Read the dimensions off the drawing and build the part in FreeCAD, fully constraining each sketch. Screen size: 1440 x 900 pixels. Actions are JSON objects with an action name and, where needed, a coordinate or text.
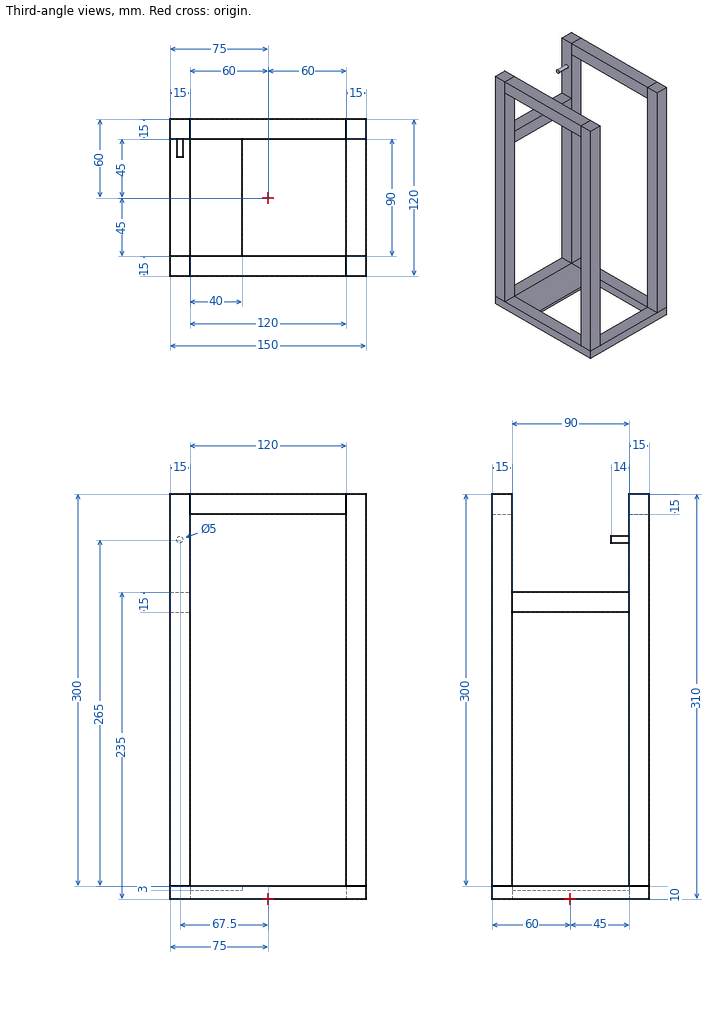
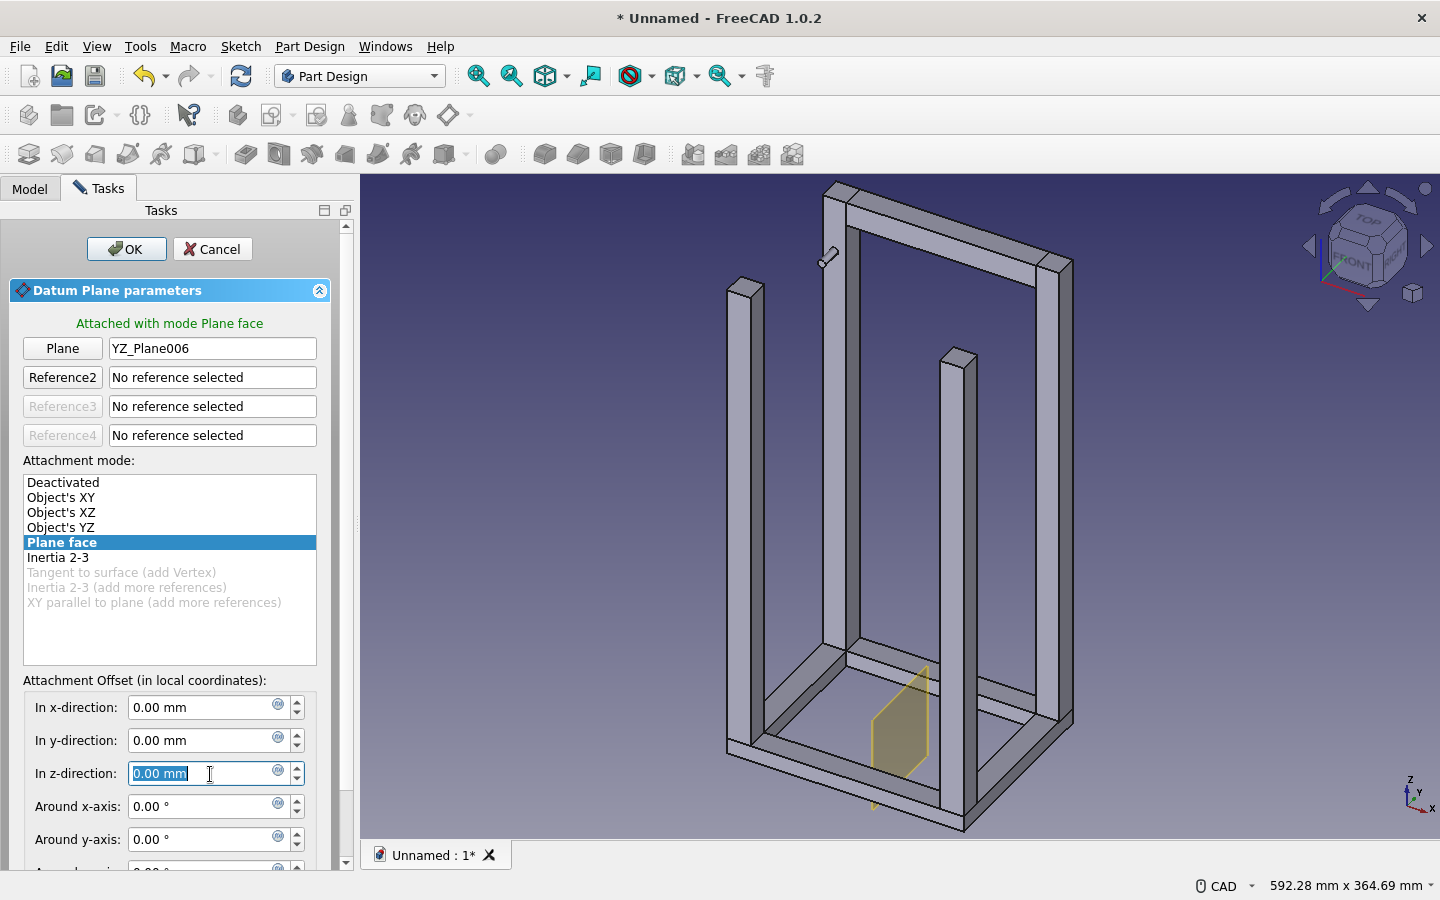
{"action": "type", "text": "-60"}
{"action": "key", "text": "Tab"}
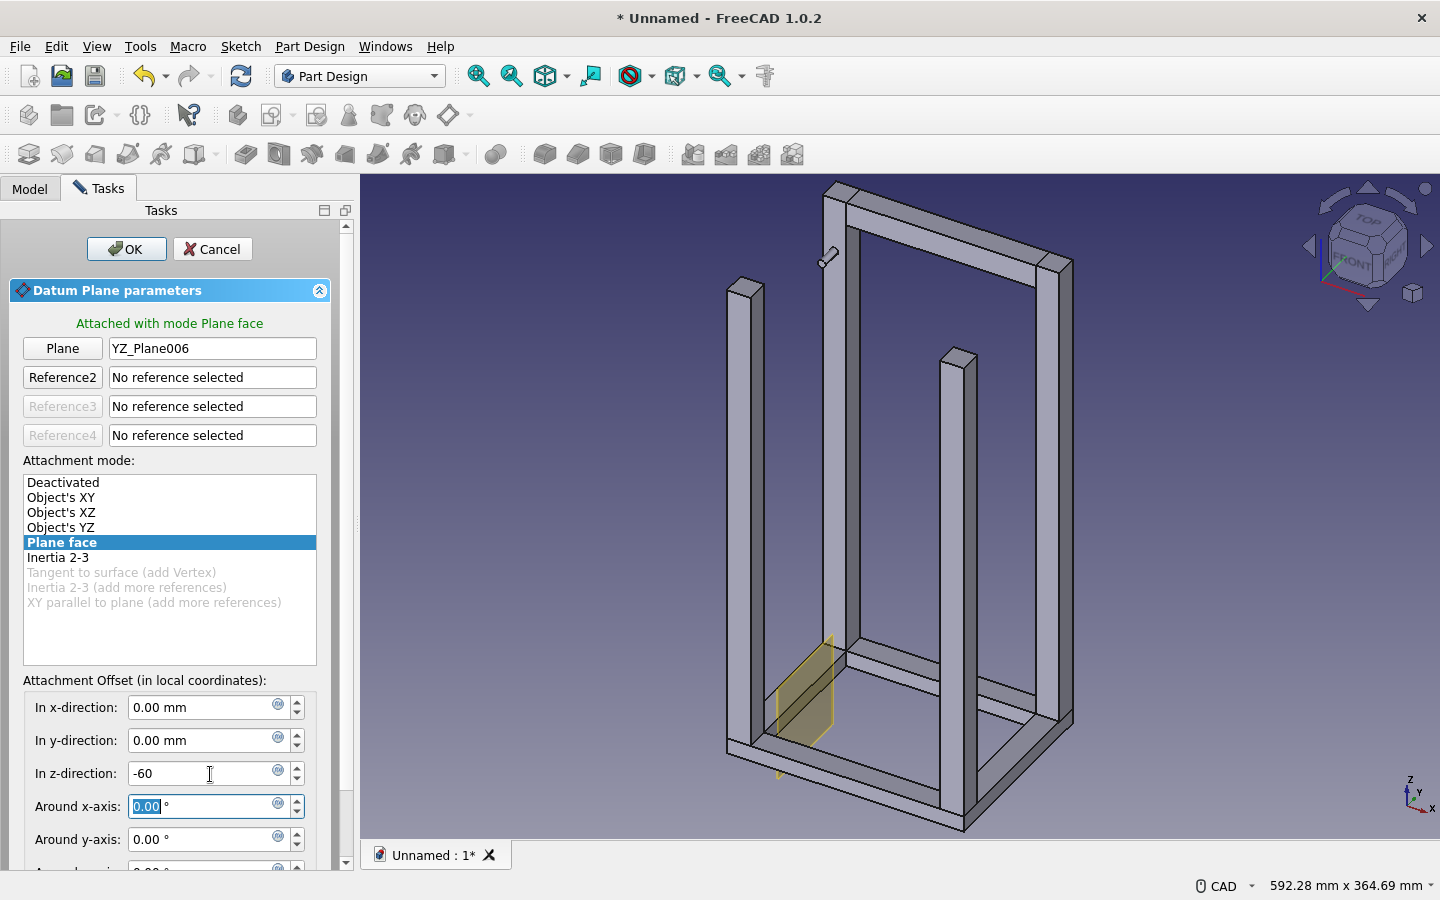
{"action": "left_click", "coordinate": [127, 249]}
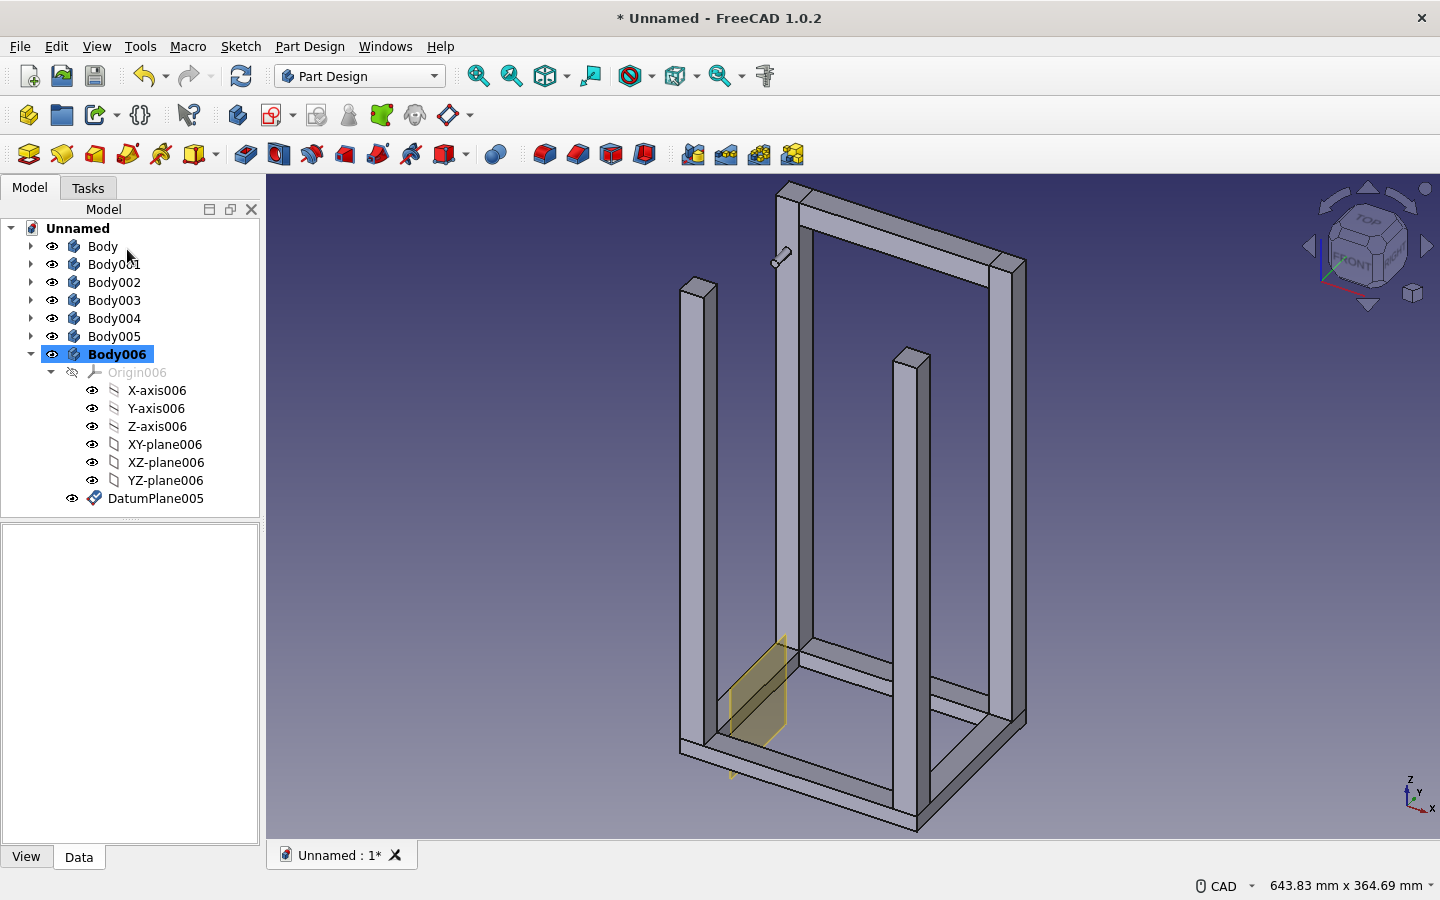
{"action": "left_click", "coordinate": [117, 498]}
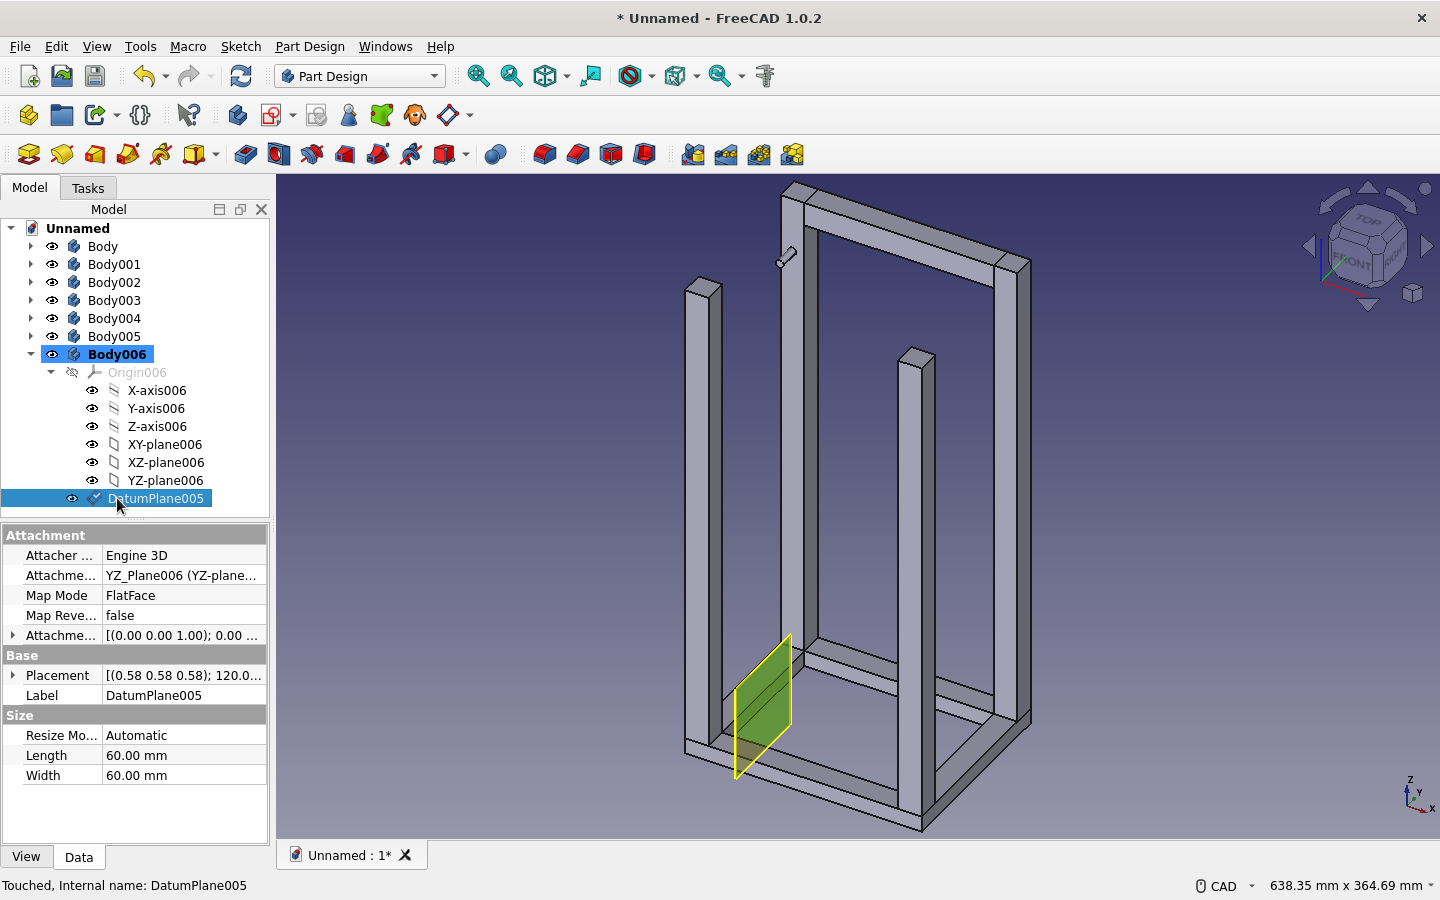
{"action": "left_click", "coordinate": [270, 116]}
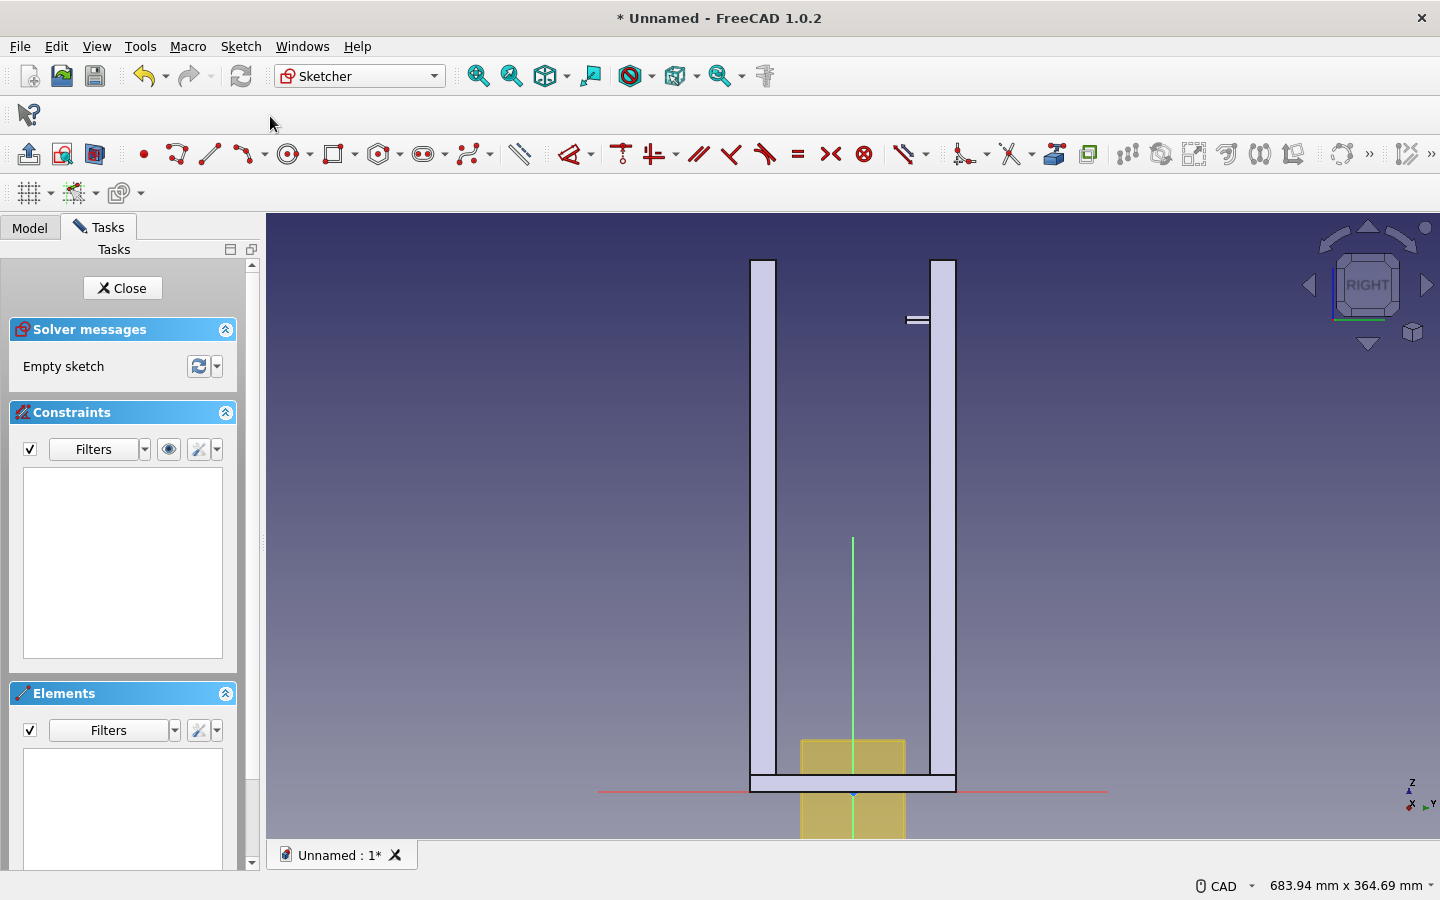
{"action": "scroll", "coordinate": [761, 256], "scroll_direction": "up", "scroll_amount": 14}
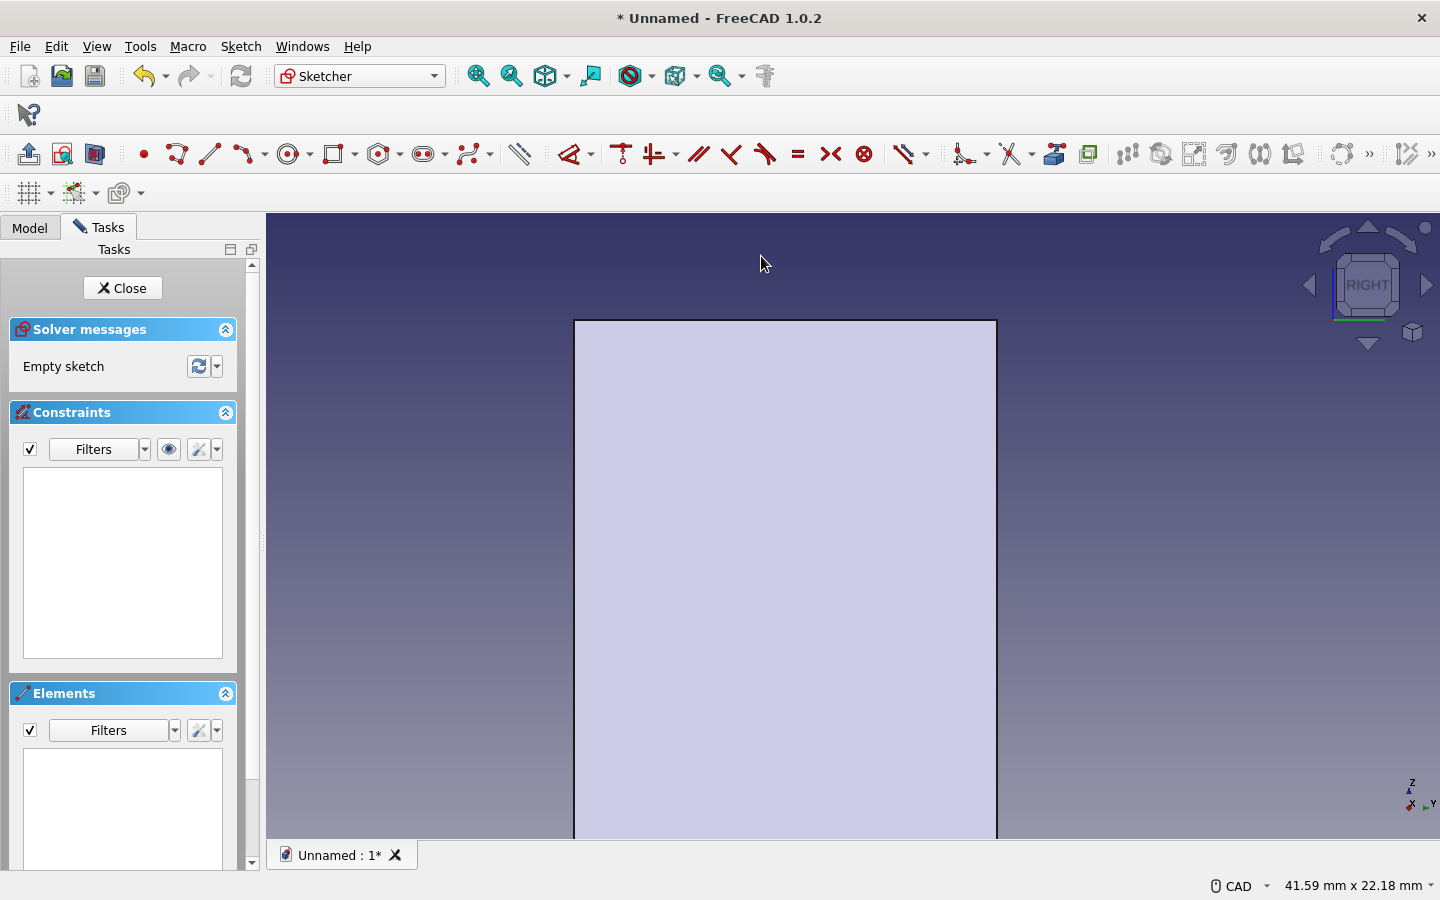
{"action": "left_click", "coordinate": [332, 154]}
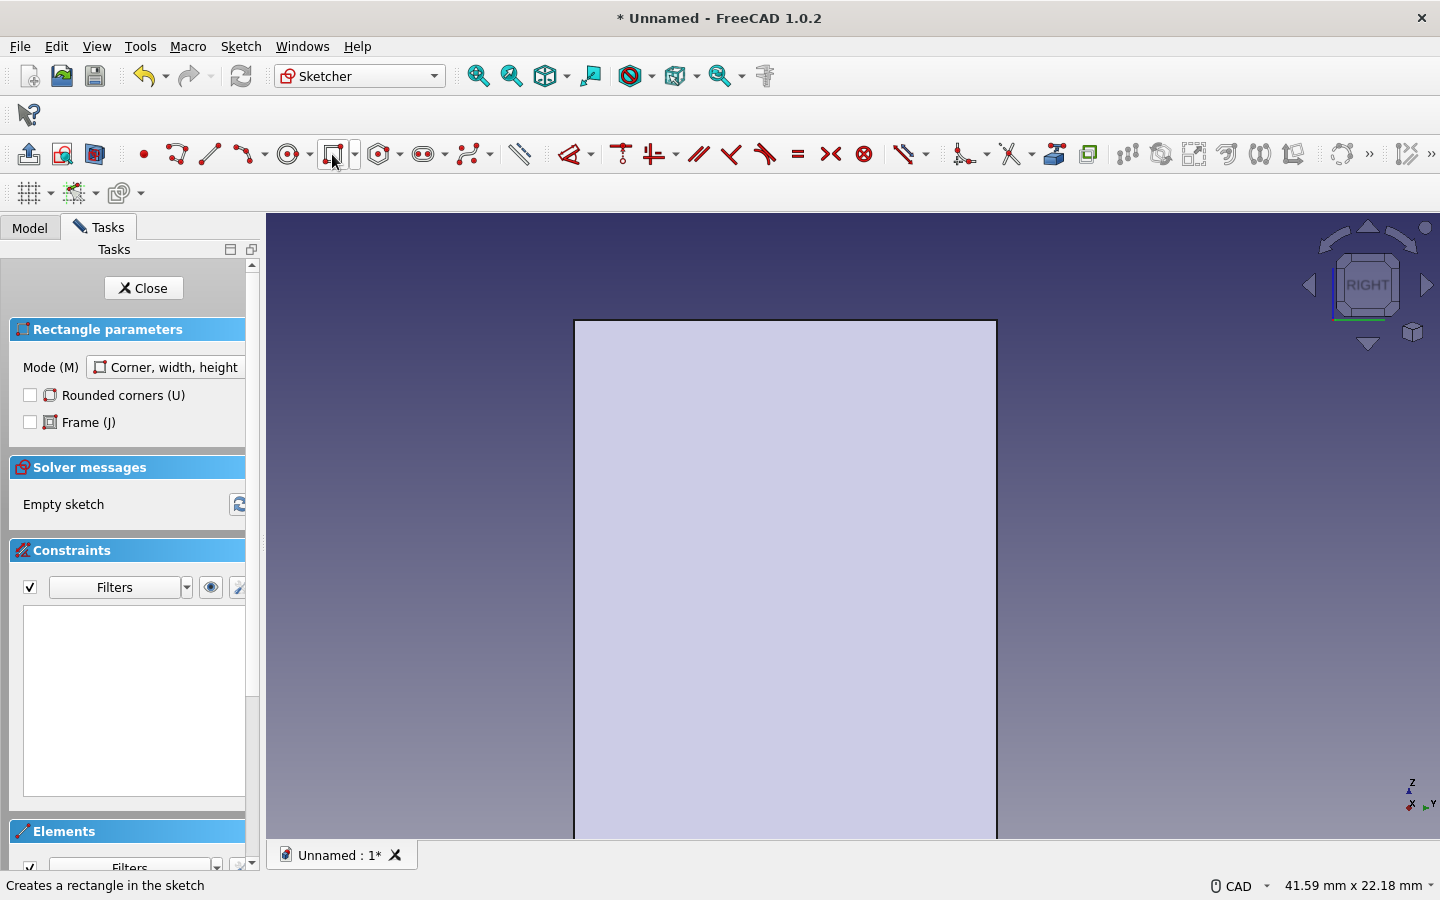
{"action": "left_click", "coordinate": [574, 320]}
{"action": "left_click", "coordinate": [997, 743]}
{"action": "key", "text": "Escape"}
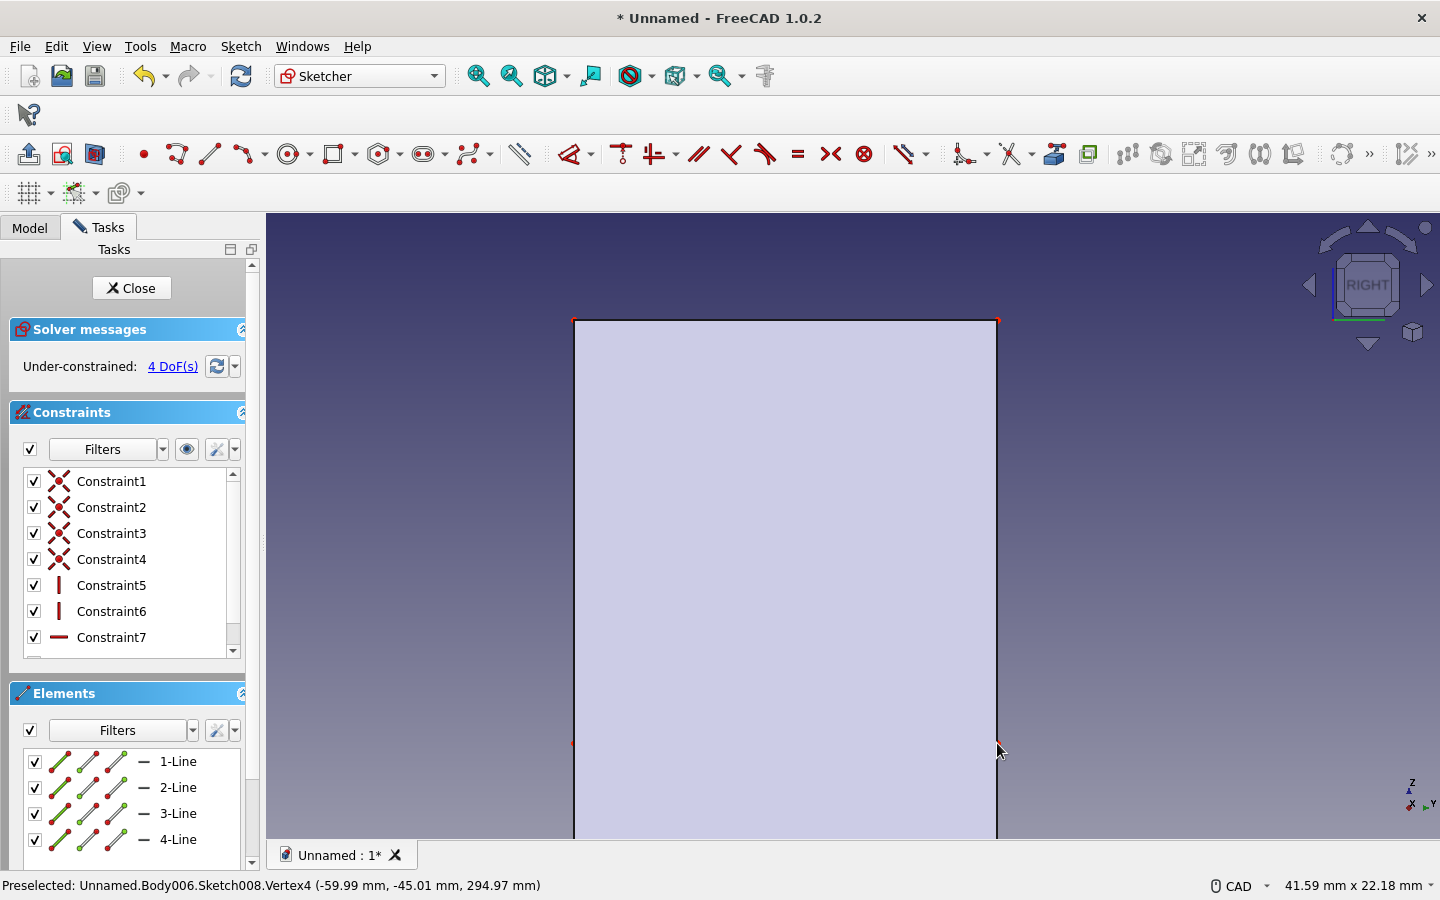
{"action": "left_click", "coordinate": [568, 154]}